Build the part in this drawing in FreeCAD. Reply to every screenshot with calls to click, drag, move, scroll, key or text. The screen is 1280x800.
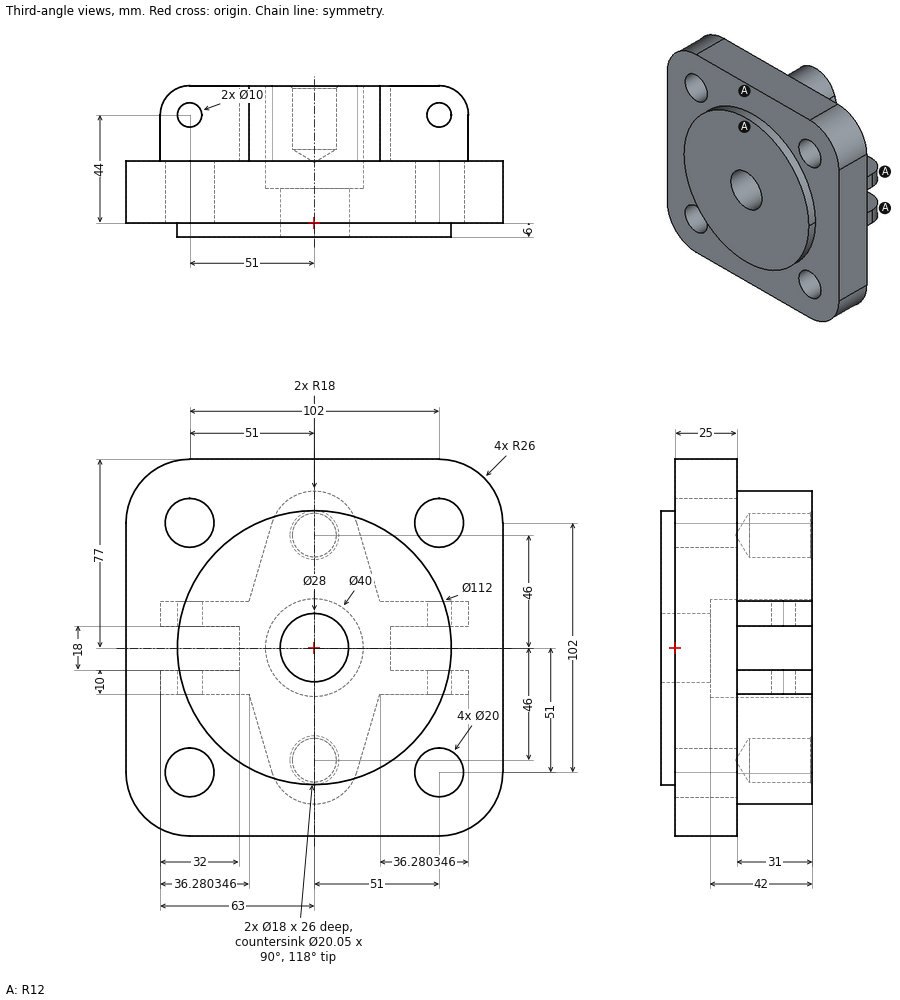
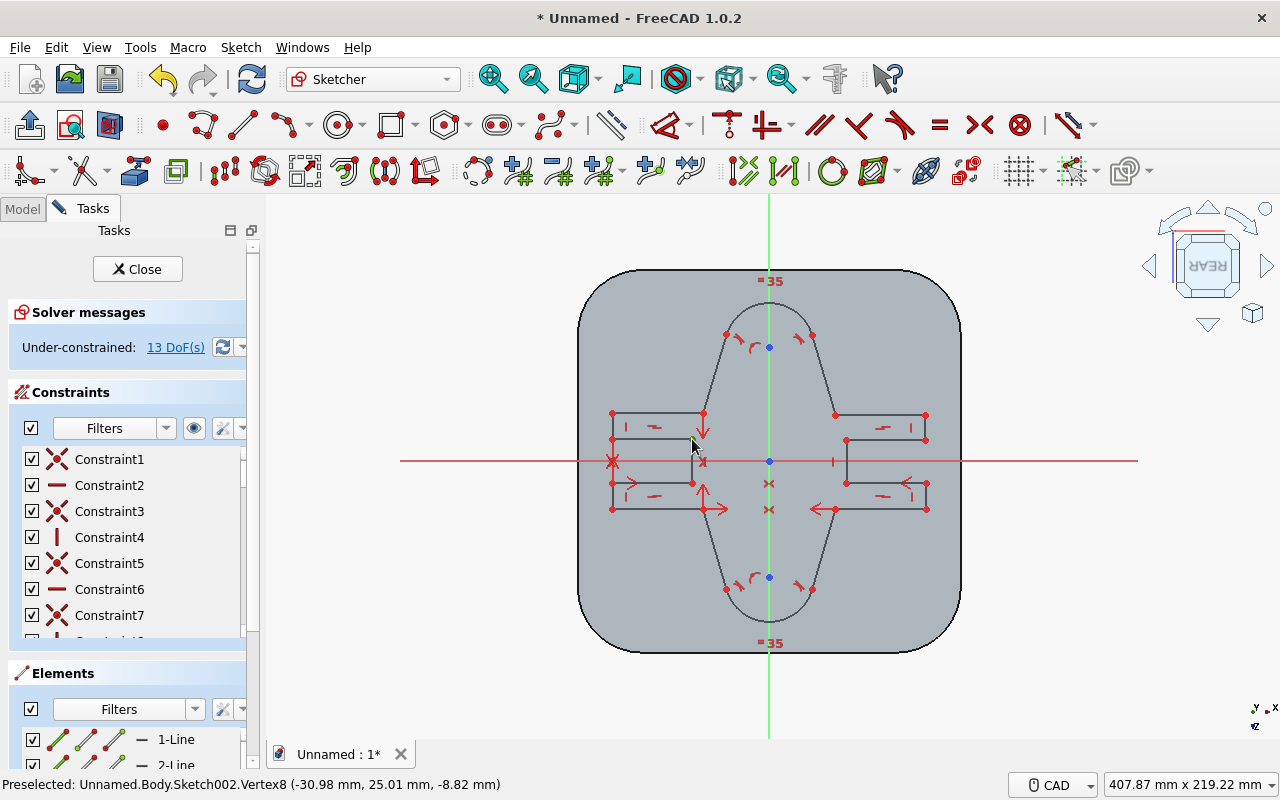
click(847, 440)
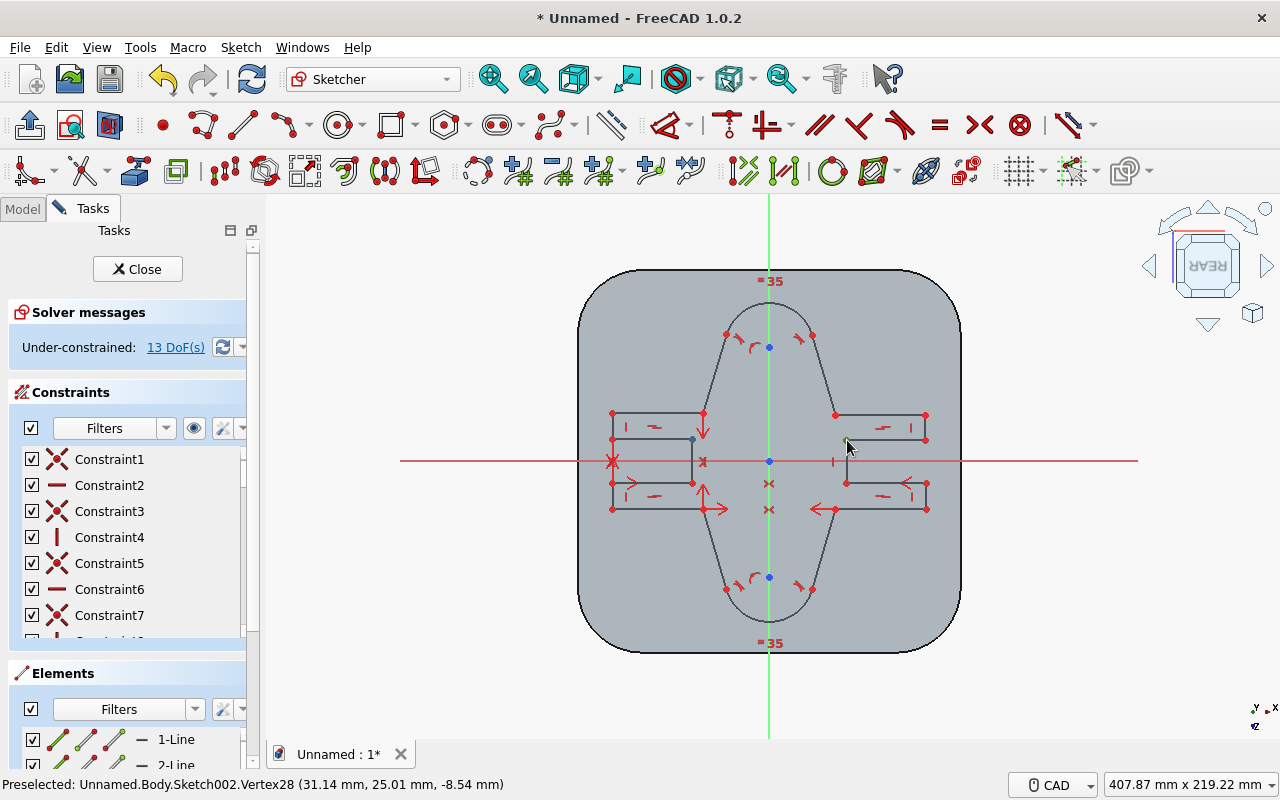
click(769, 676)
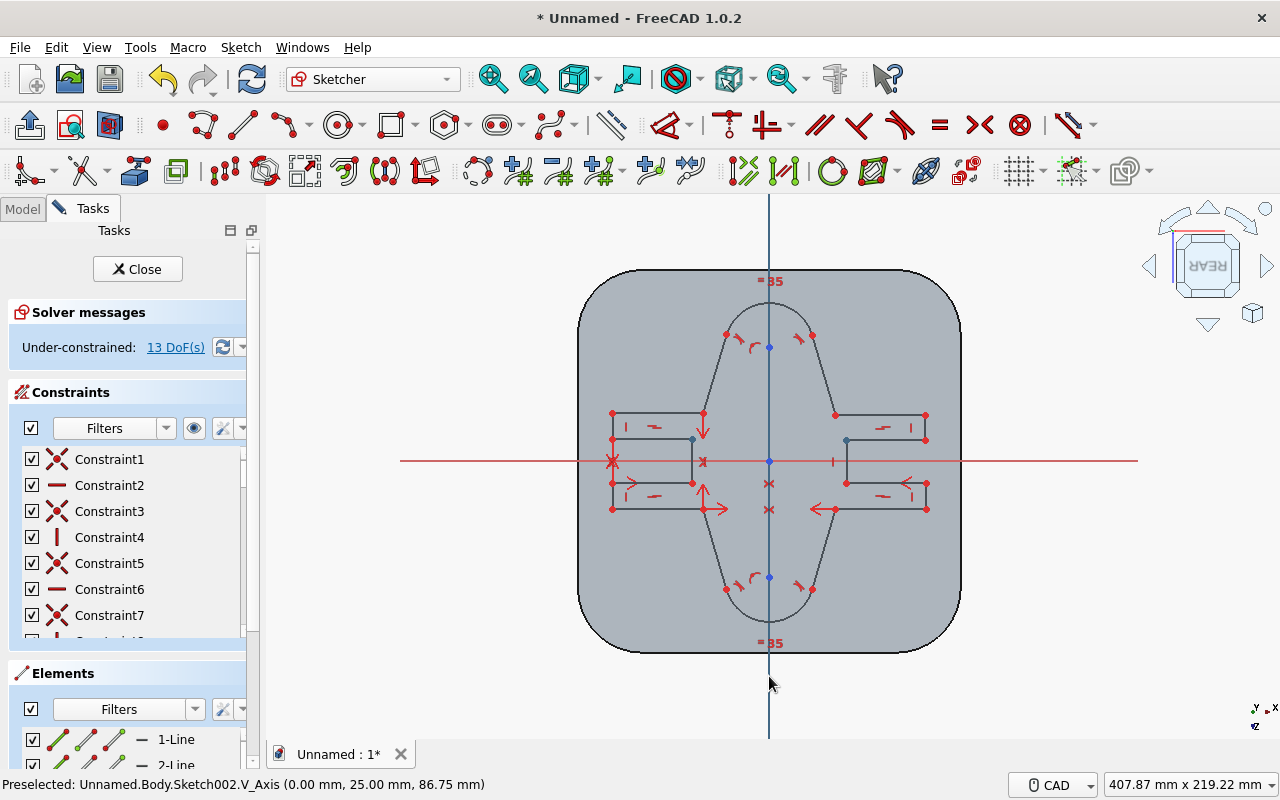
key(s)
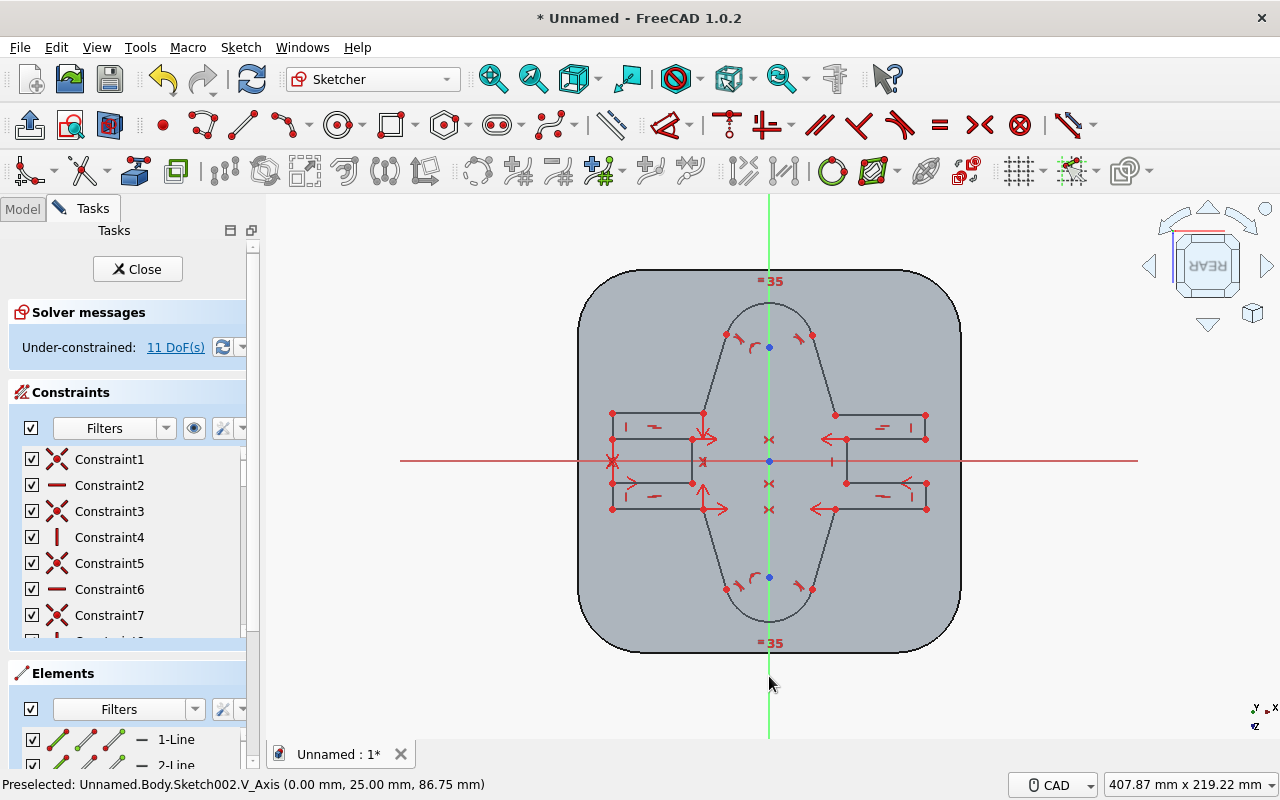
click(613, 413)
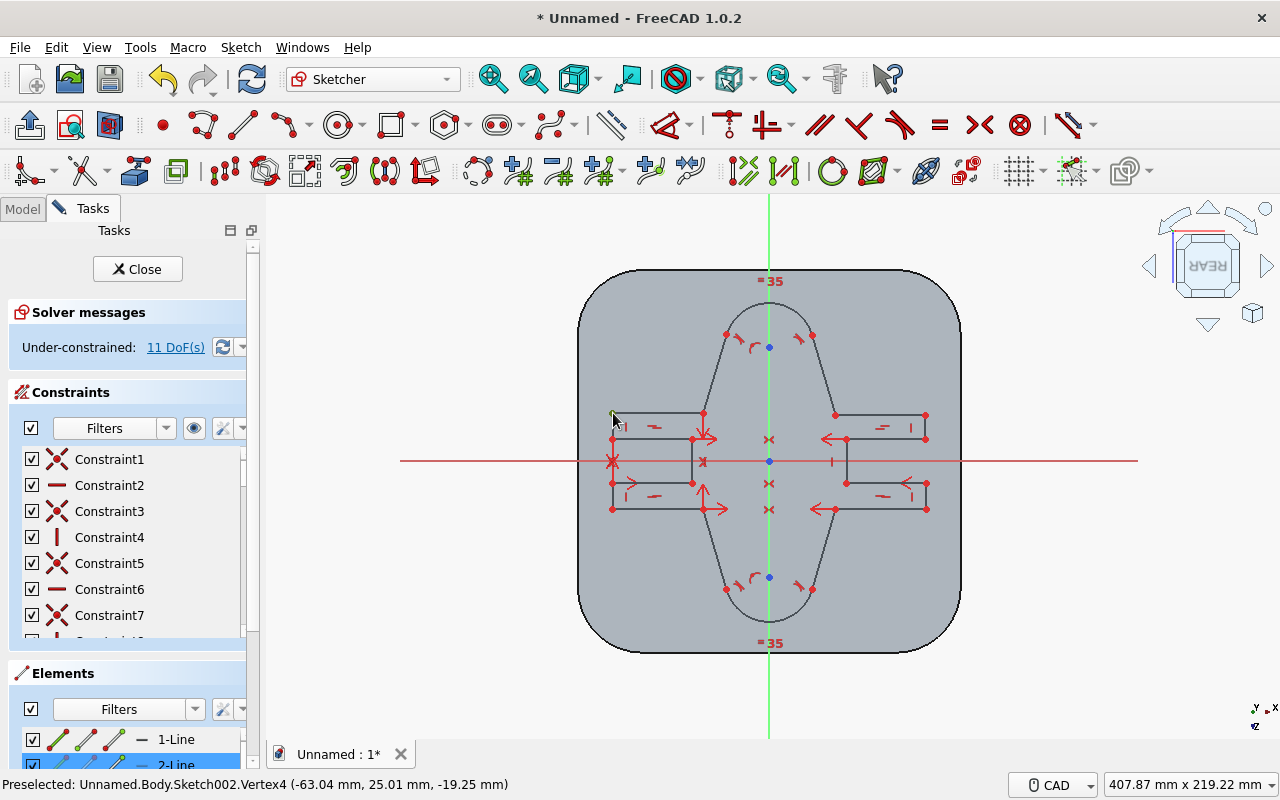
click(925, 415)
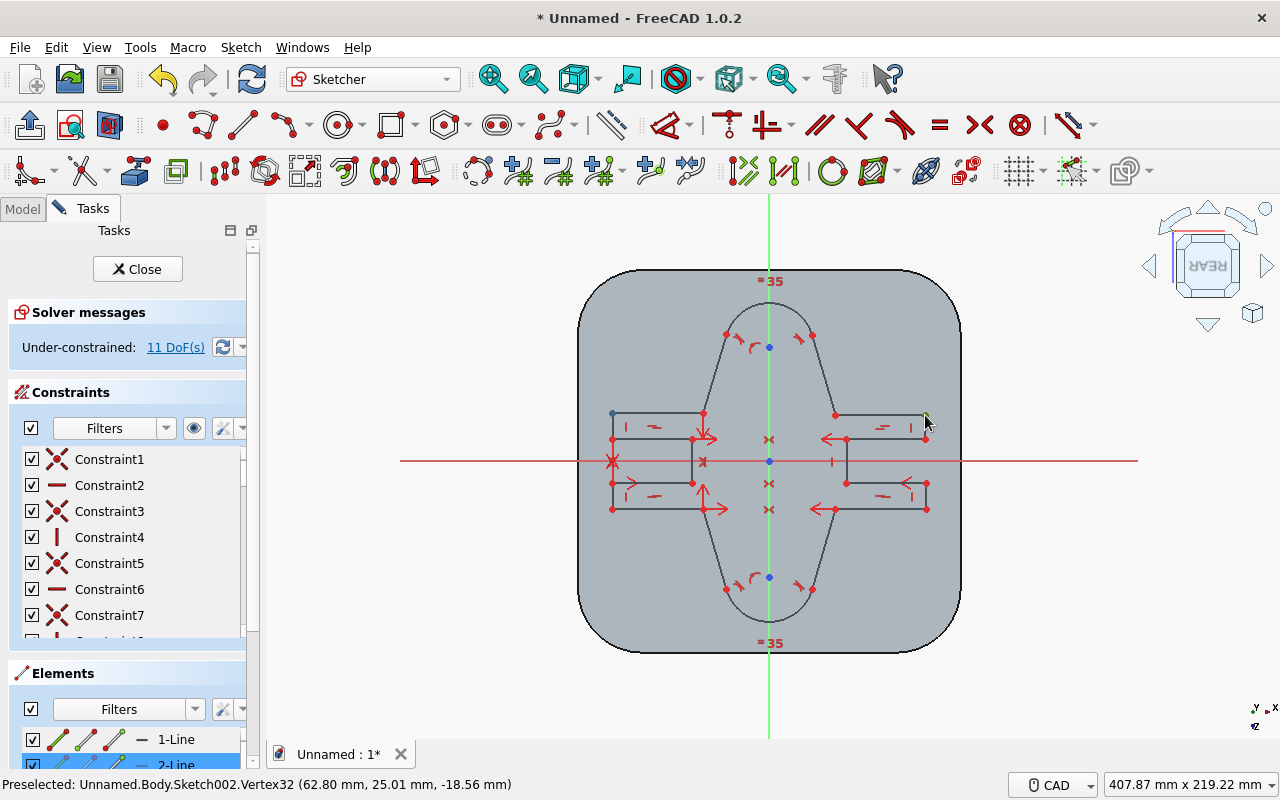
click(769, 676)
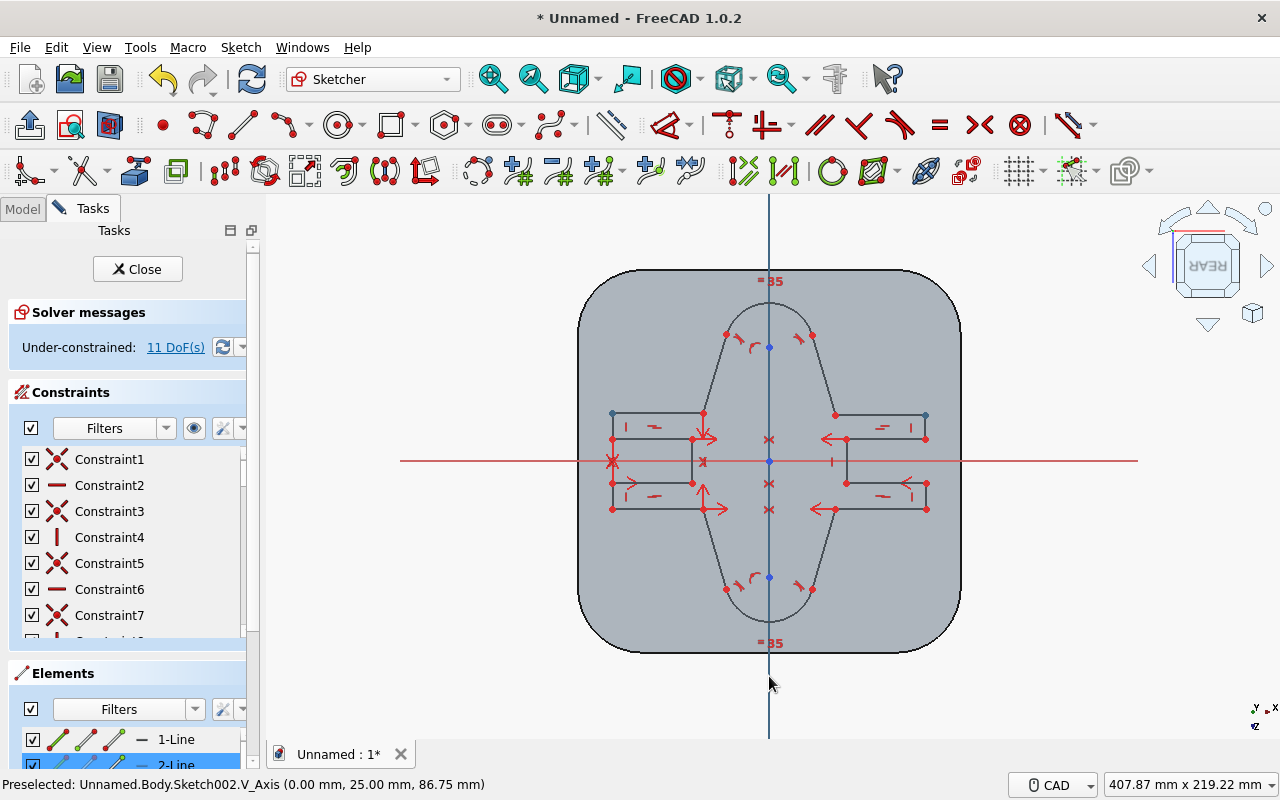
key(s)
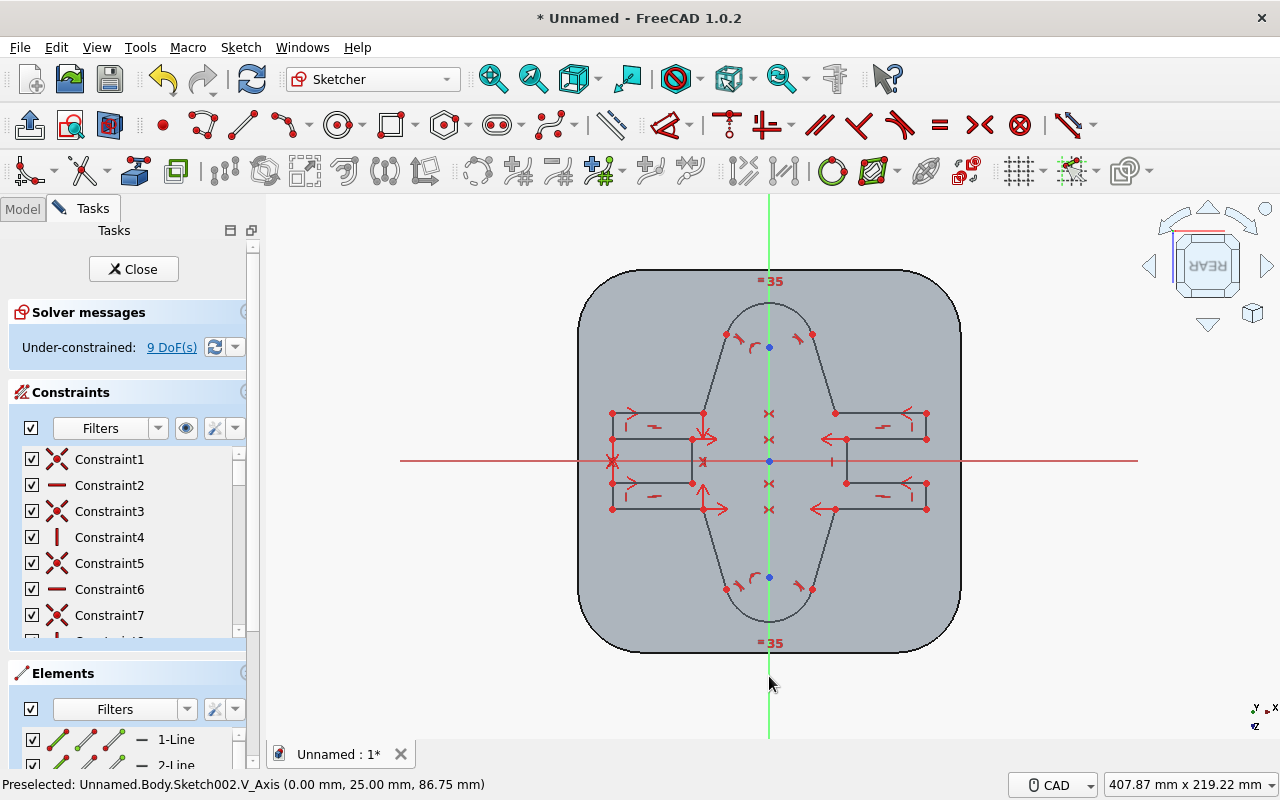
key(d)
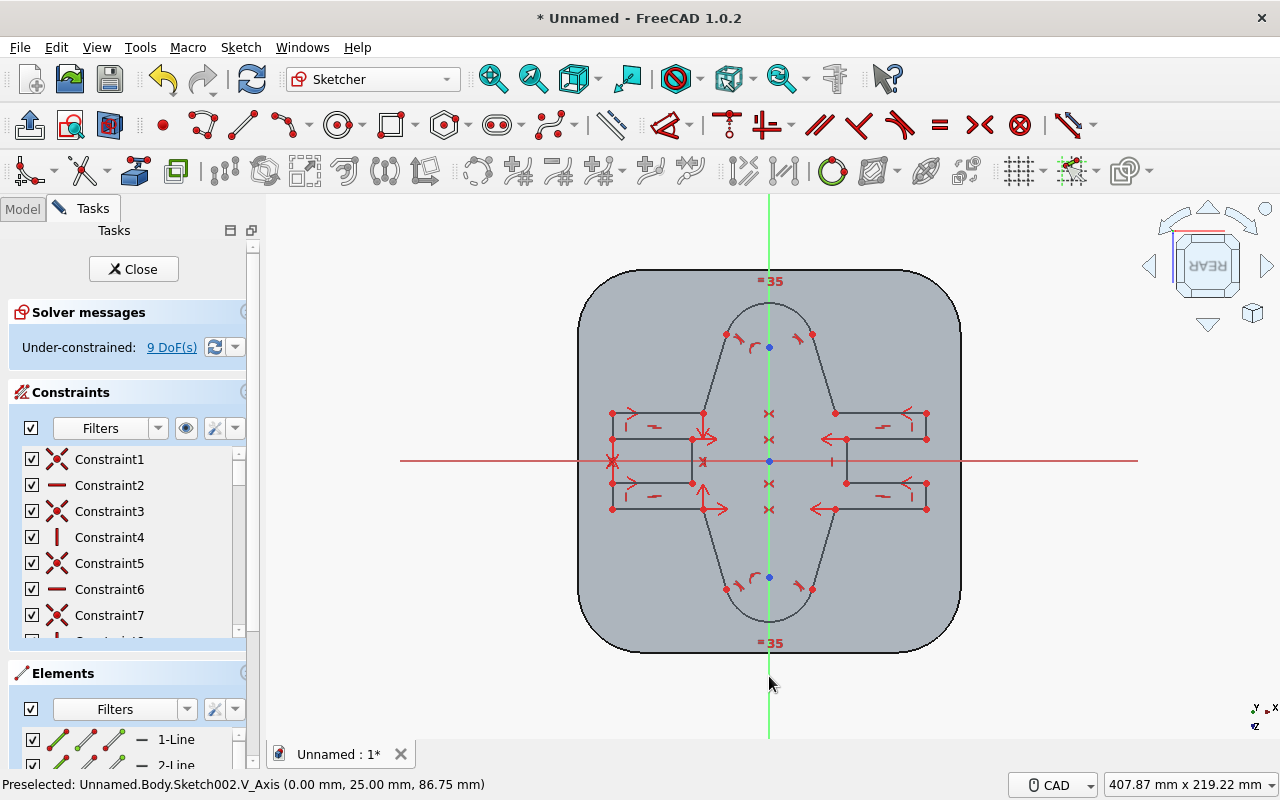
click(747, 616)
click(731, 644)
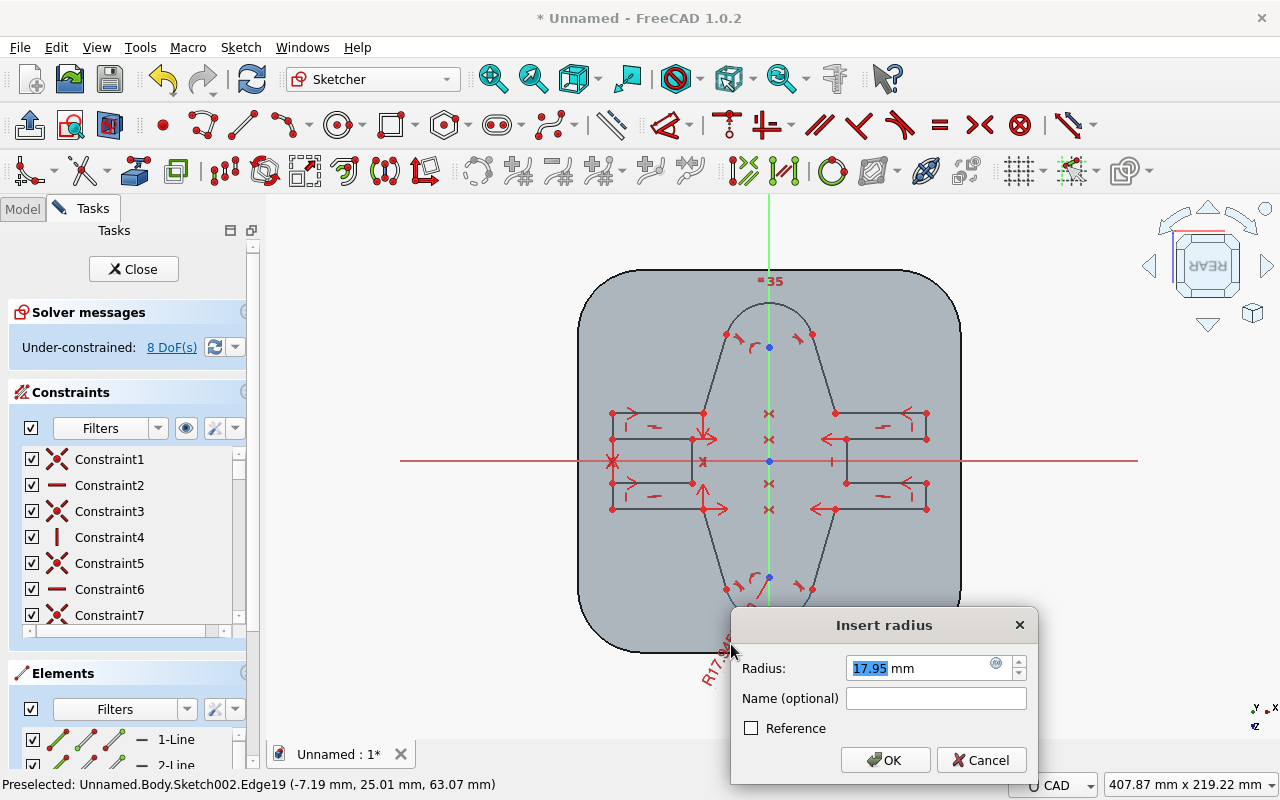
text(18)
key(Return)